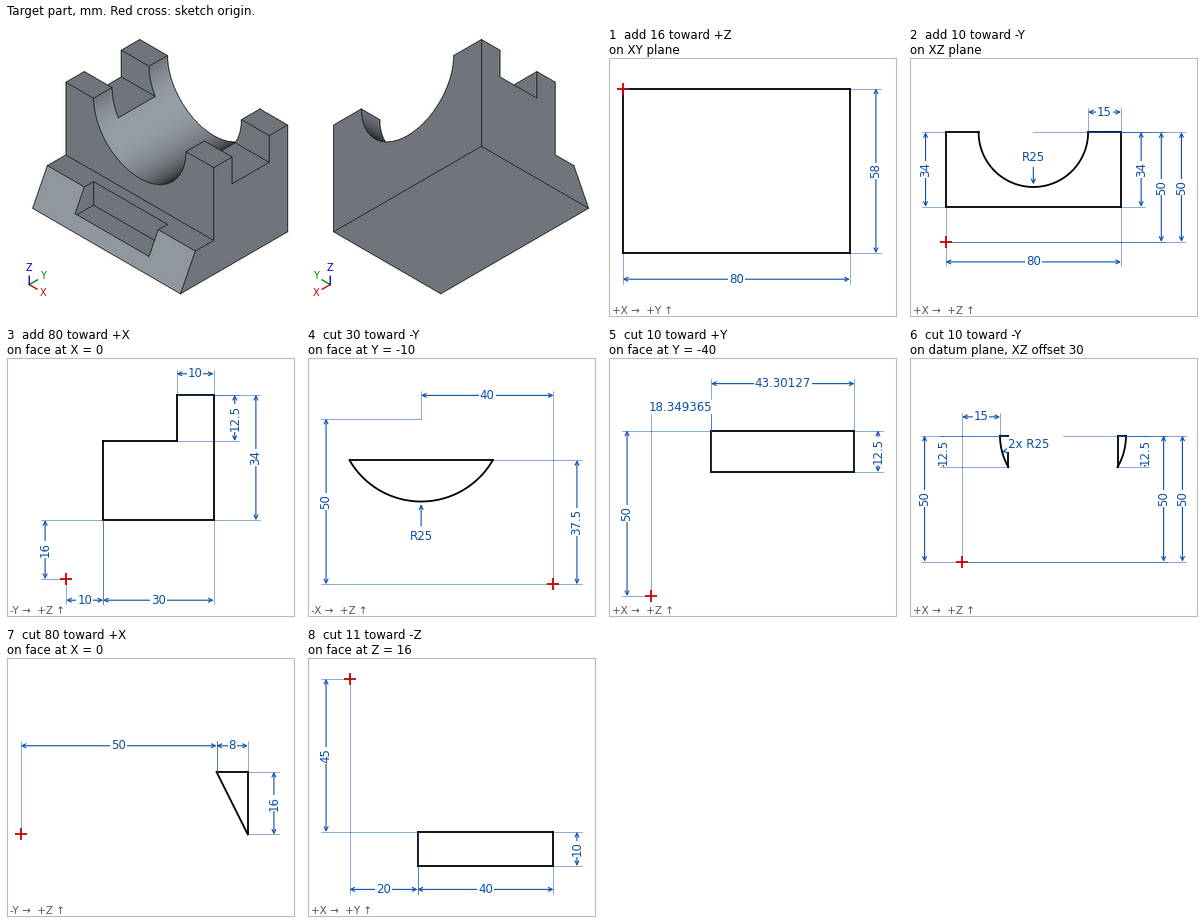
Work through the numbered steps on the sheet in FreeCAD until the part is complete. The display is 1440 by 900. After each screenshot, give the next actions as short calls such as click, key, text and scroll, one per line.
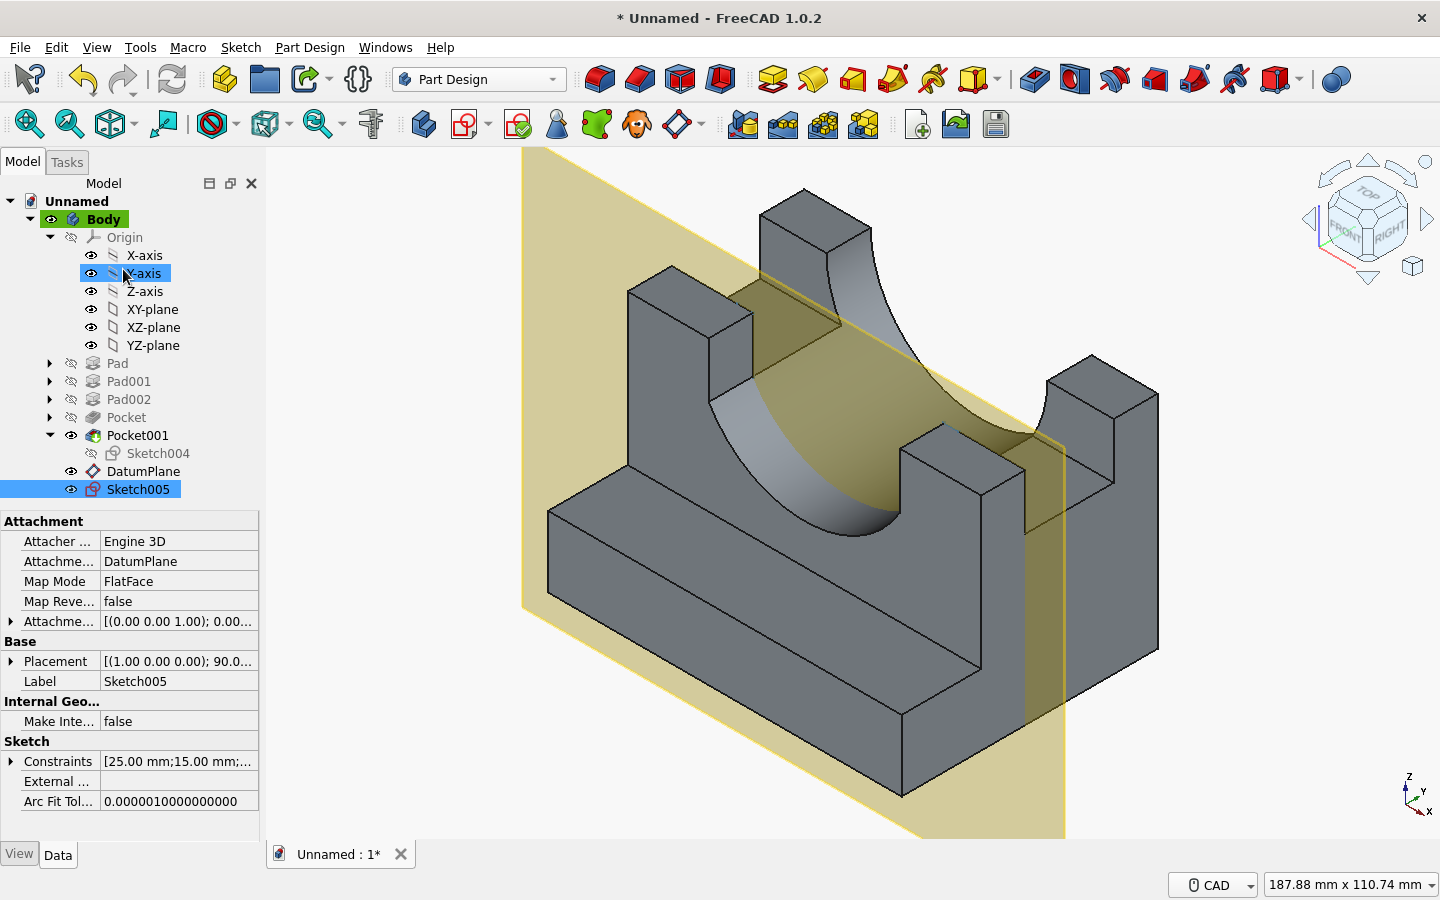
click(1036, 80)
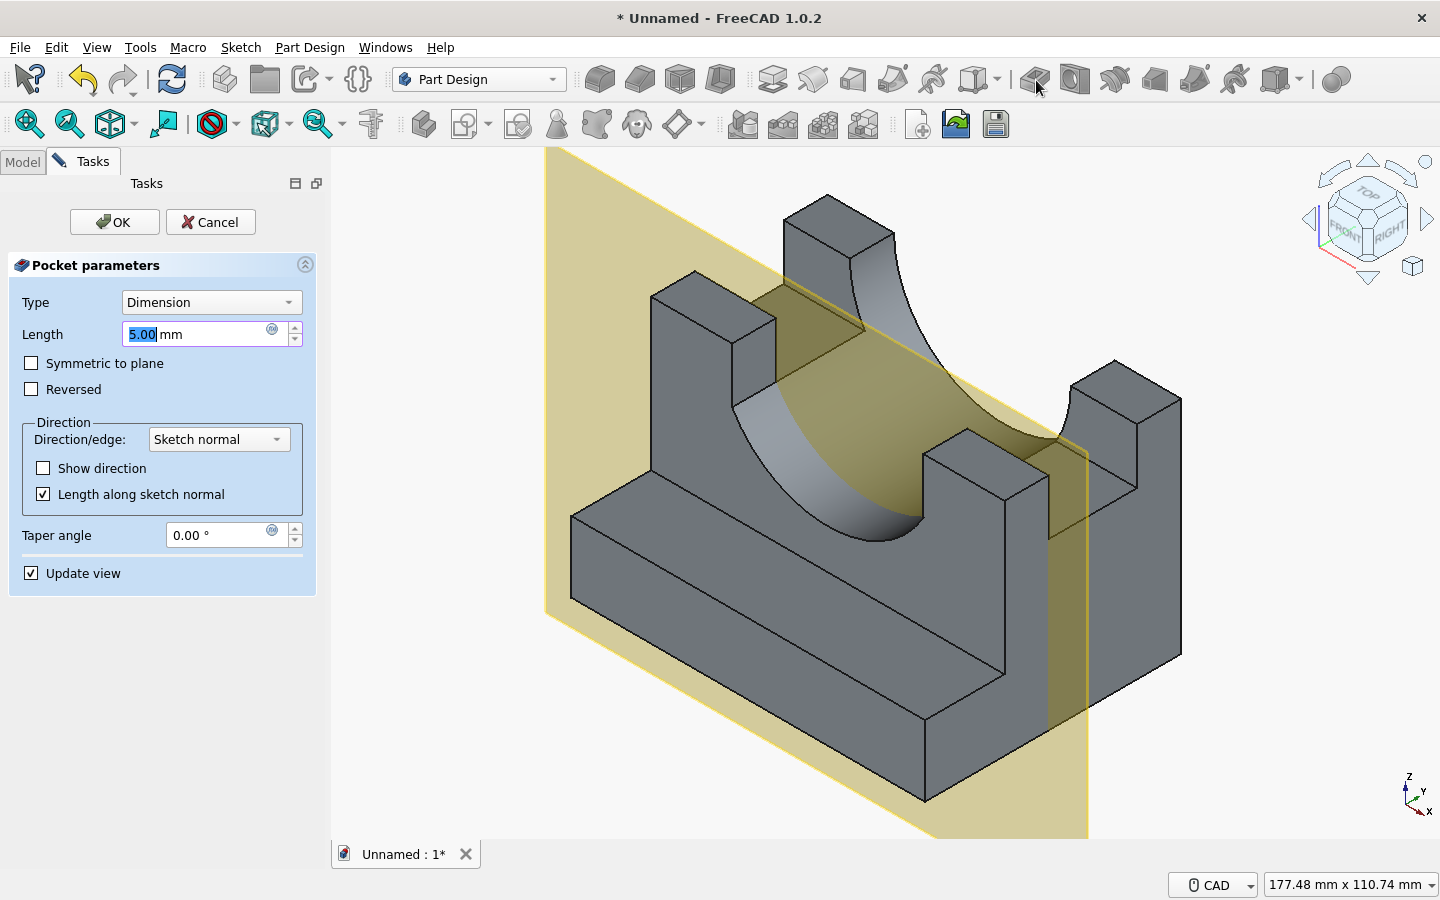
text(10)
key(Tab)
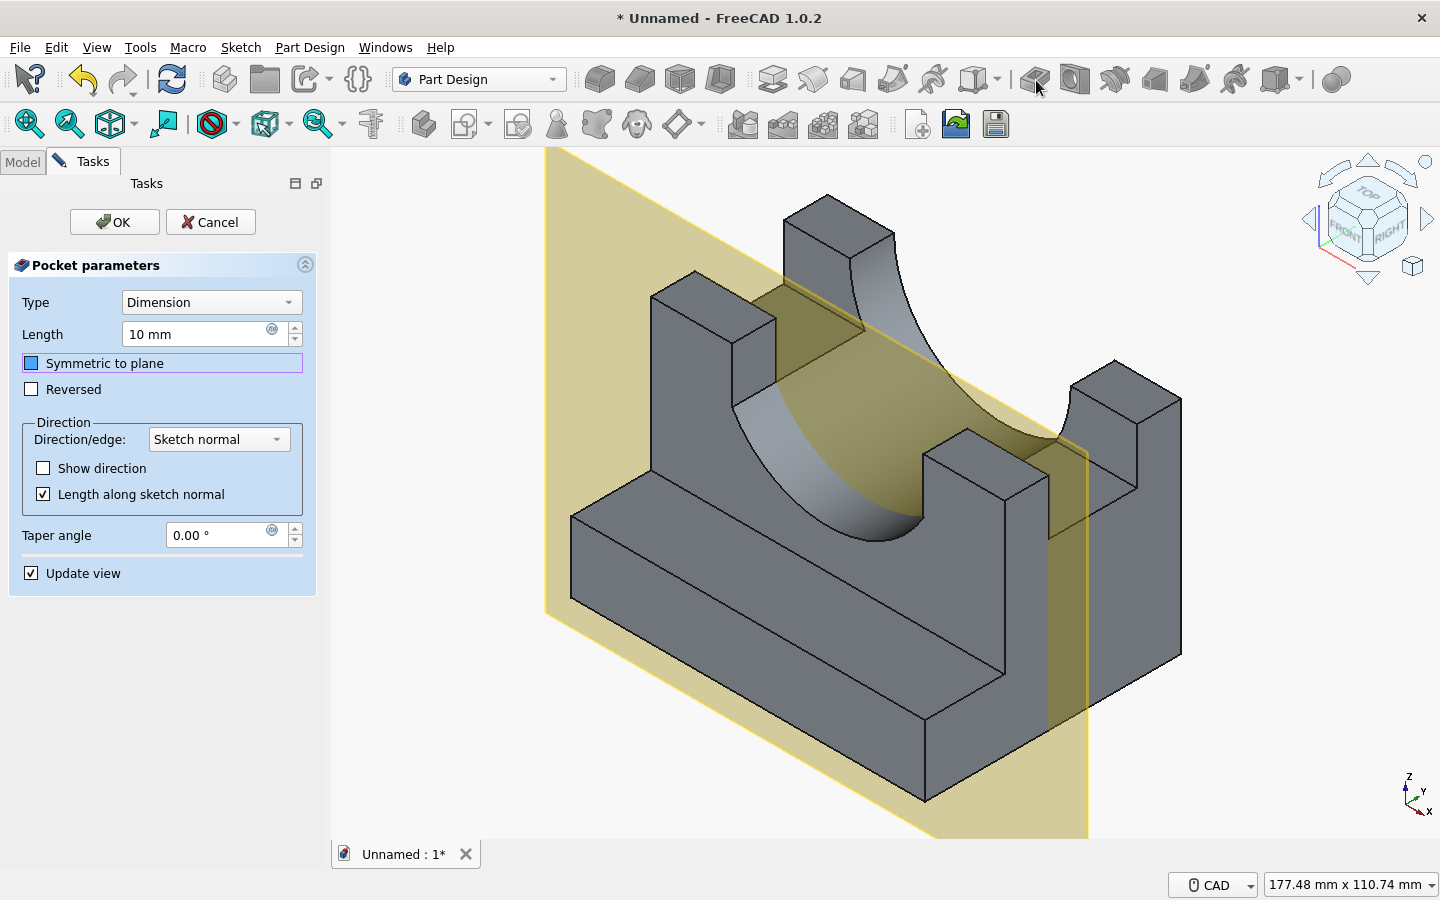
click(30, 389)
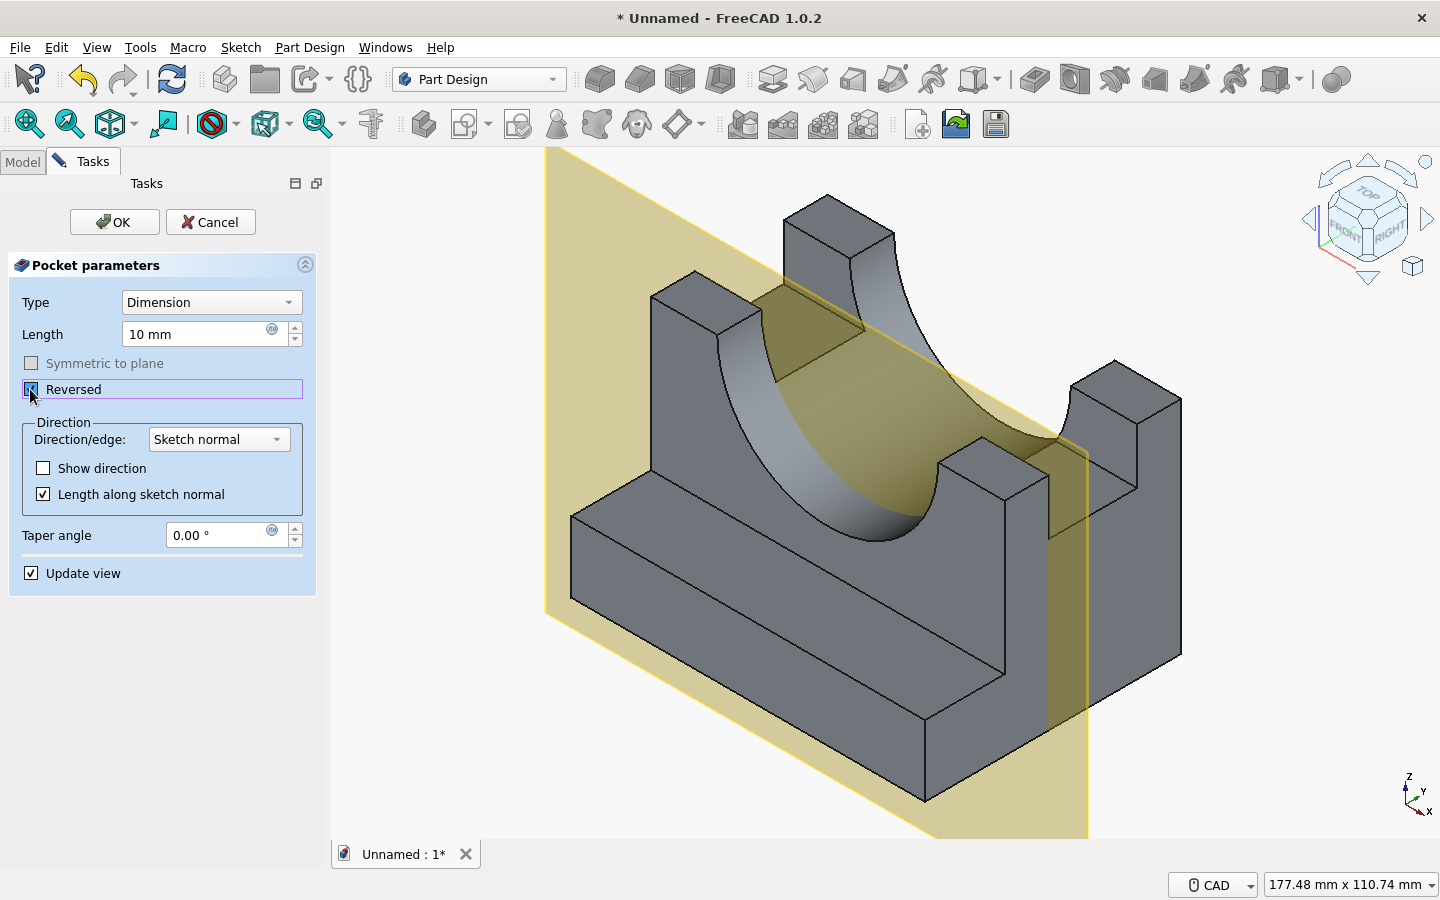
click(115, 222)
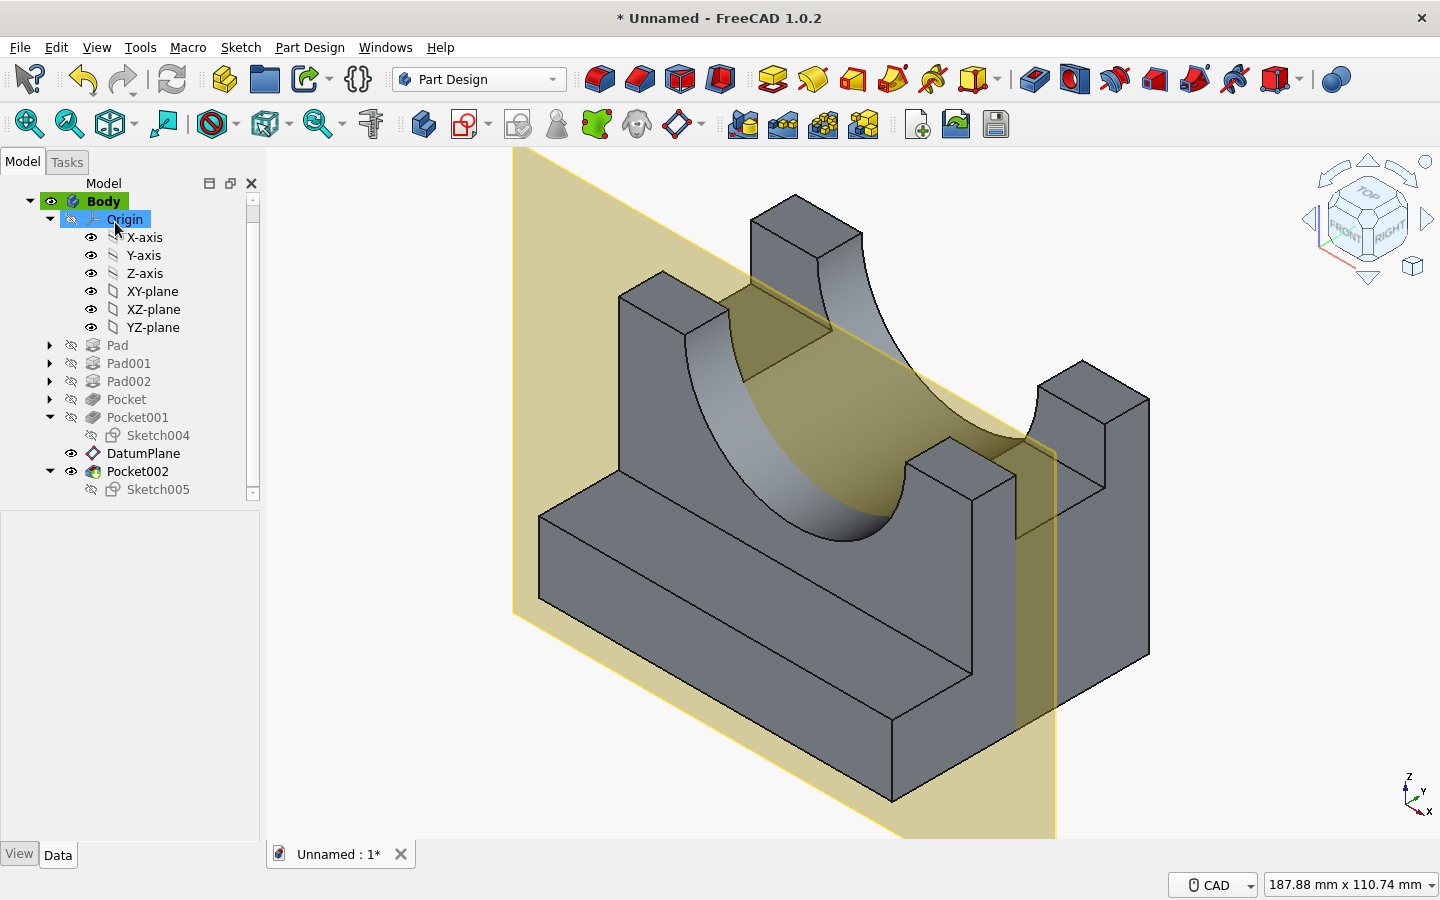
click(116, 453)
key(space)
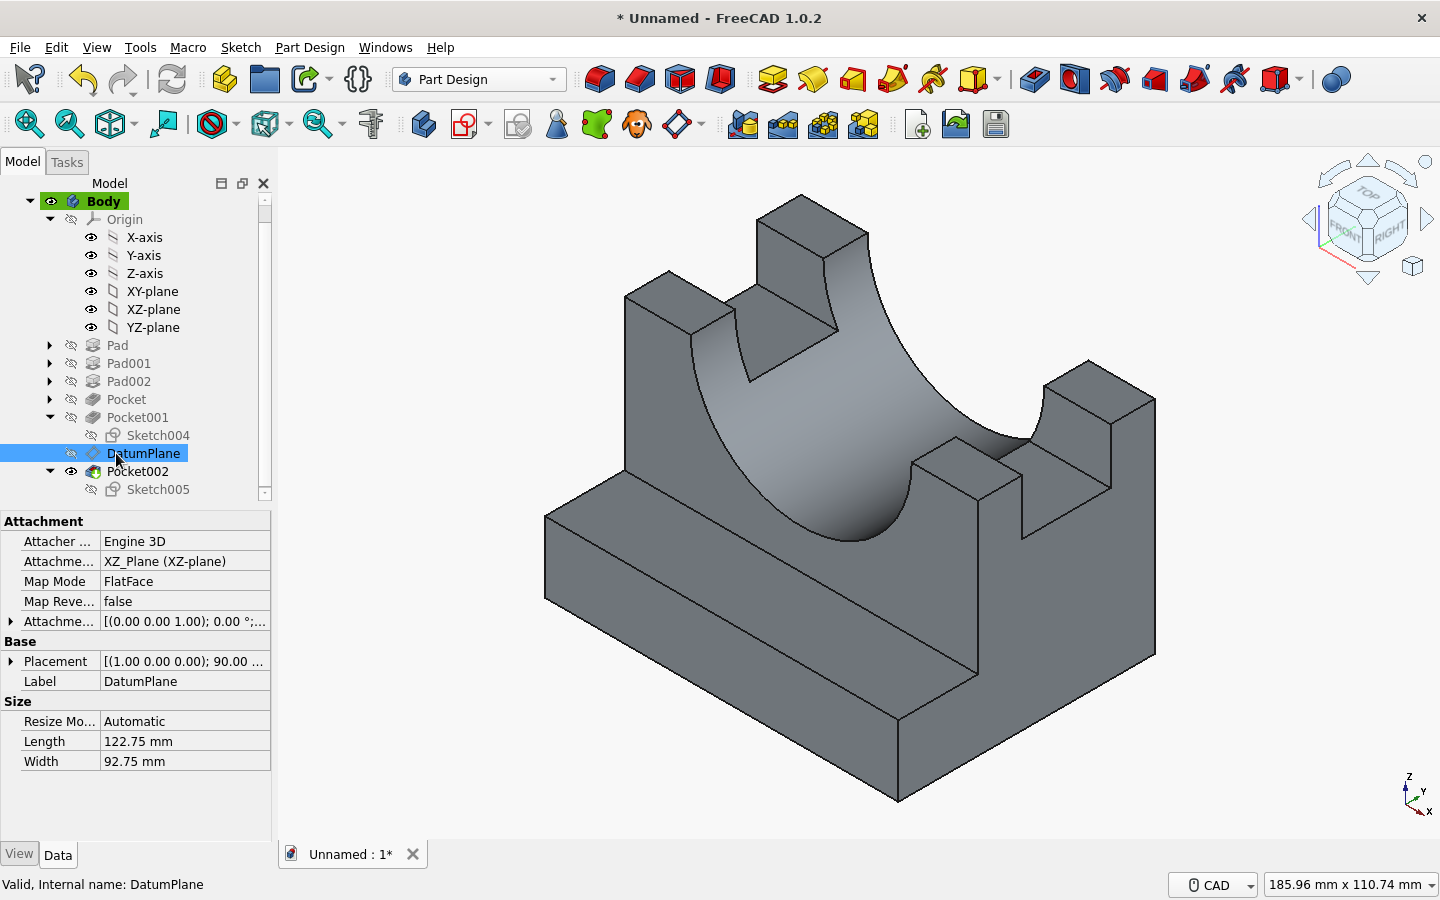
key(6)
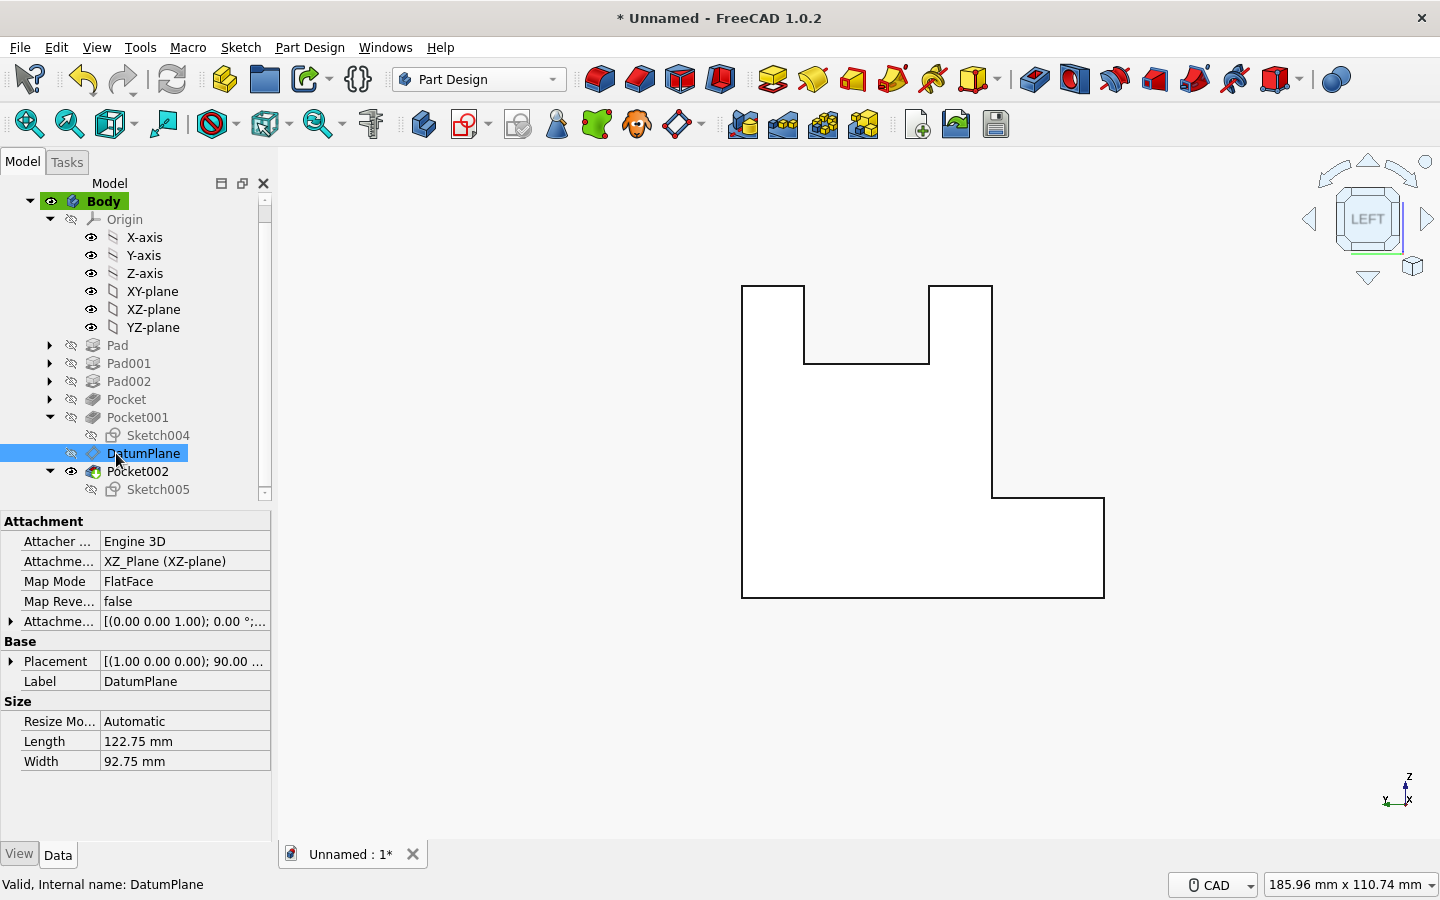
click(871, 486)